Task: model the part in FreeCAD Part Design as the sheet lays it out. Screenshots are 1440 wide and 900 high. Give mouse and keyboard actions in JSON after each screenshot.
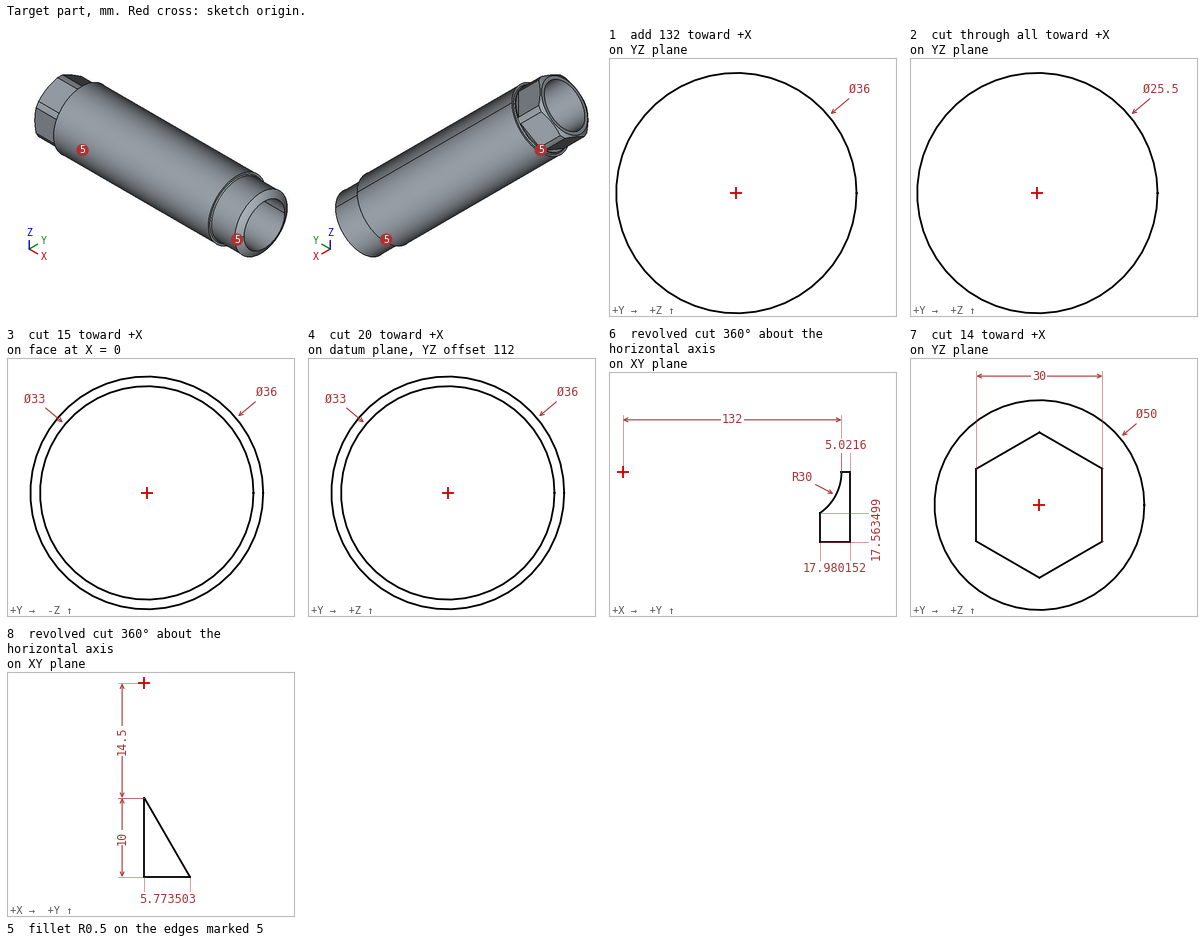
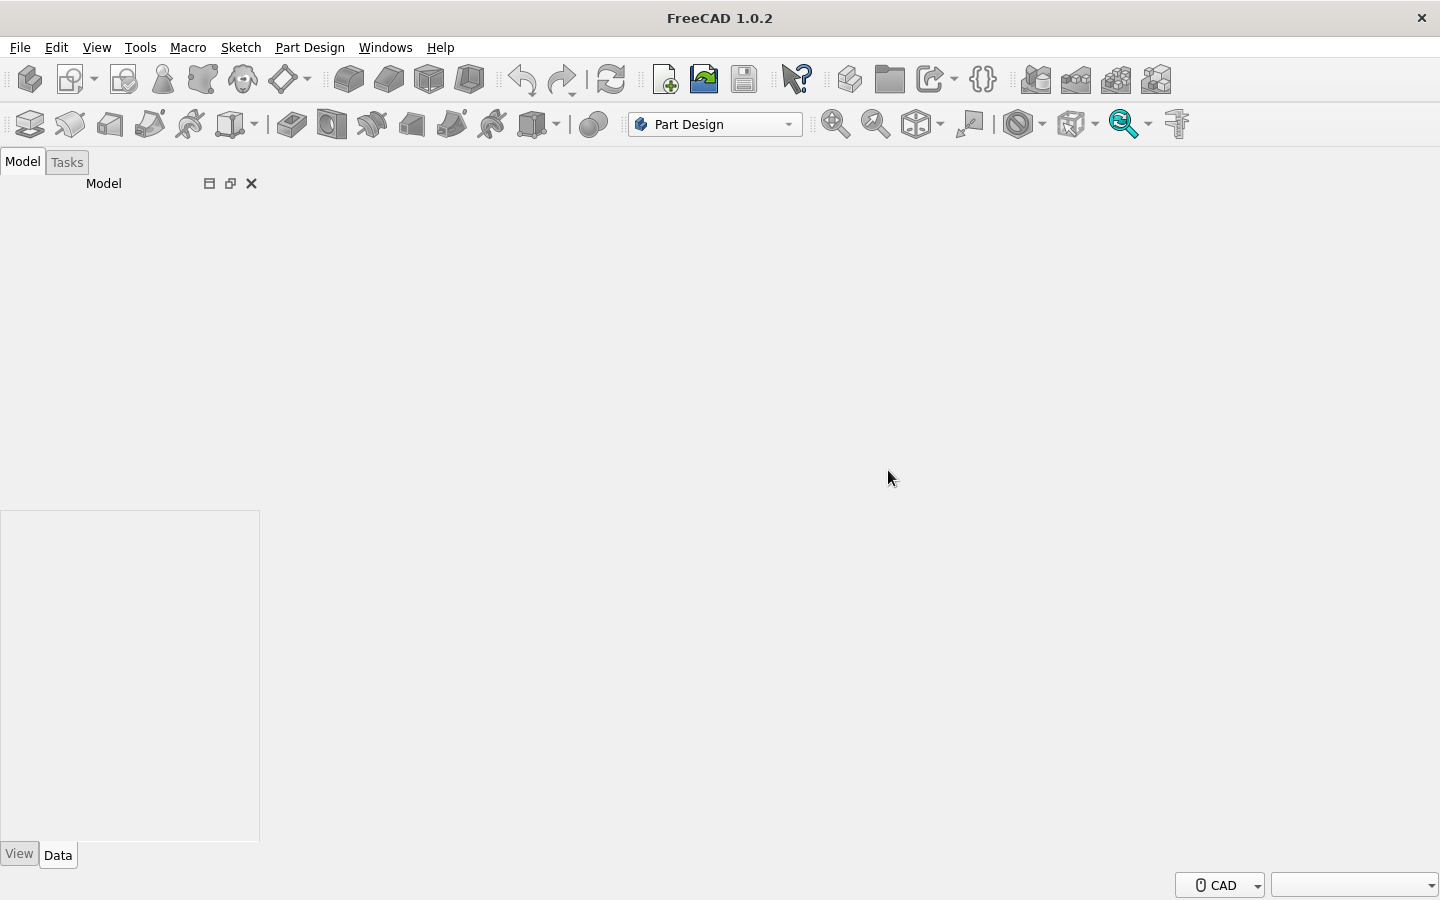
{"action": "left_click", "coordinate": [664, 80]}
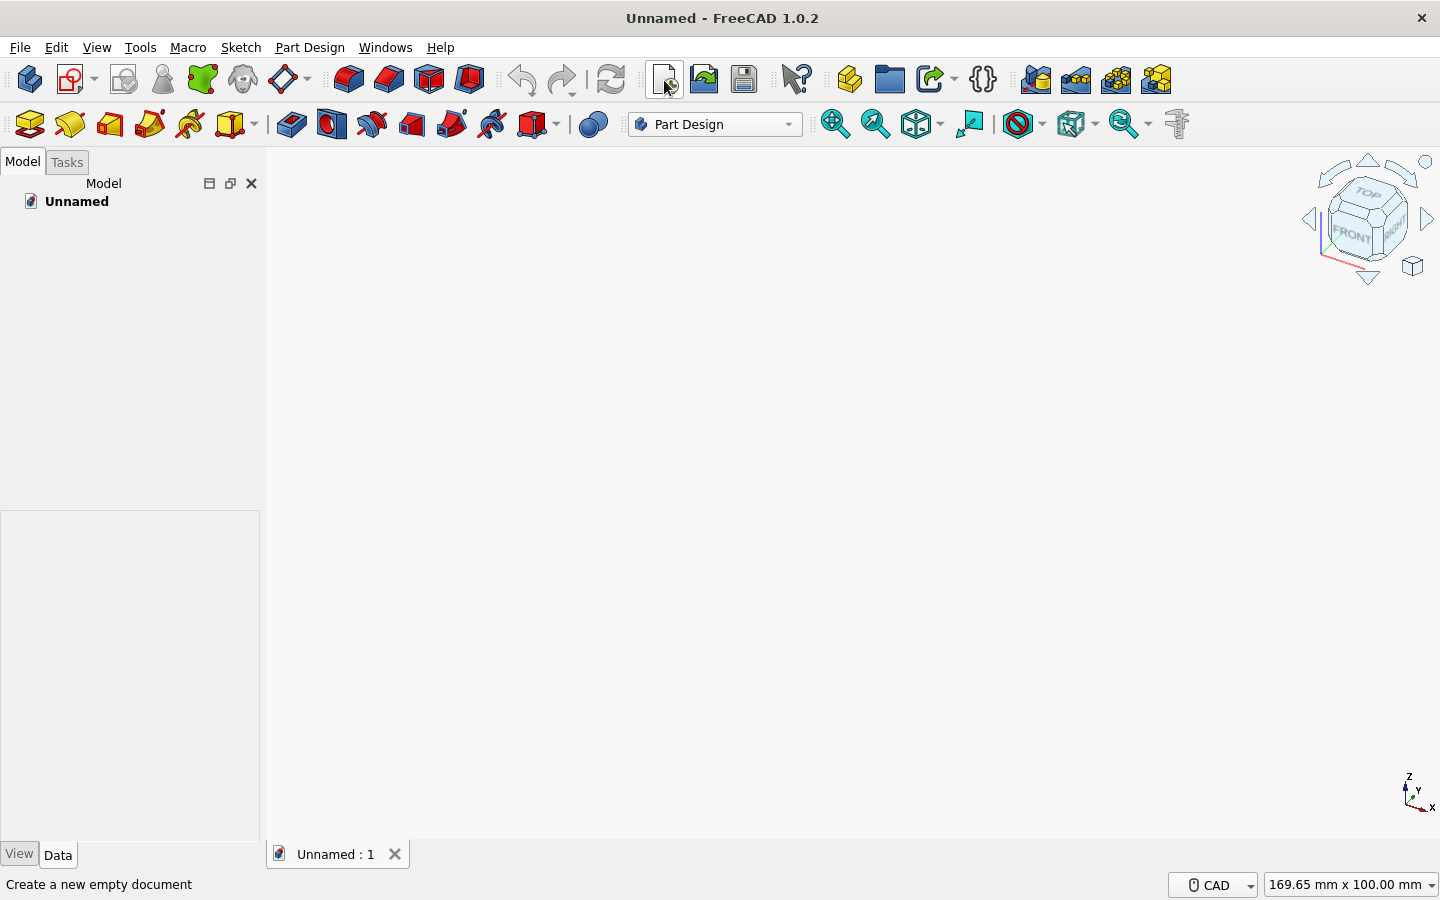
{"action": "left_click", "coordinate": [70, 80]}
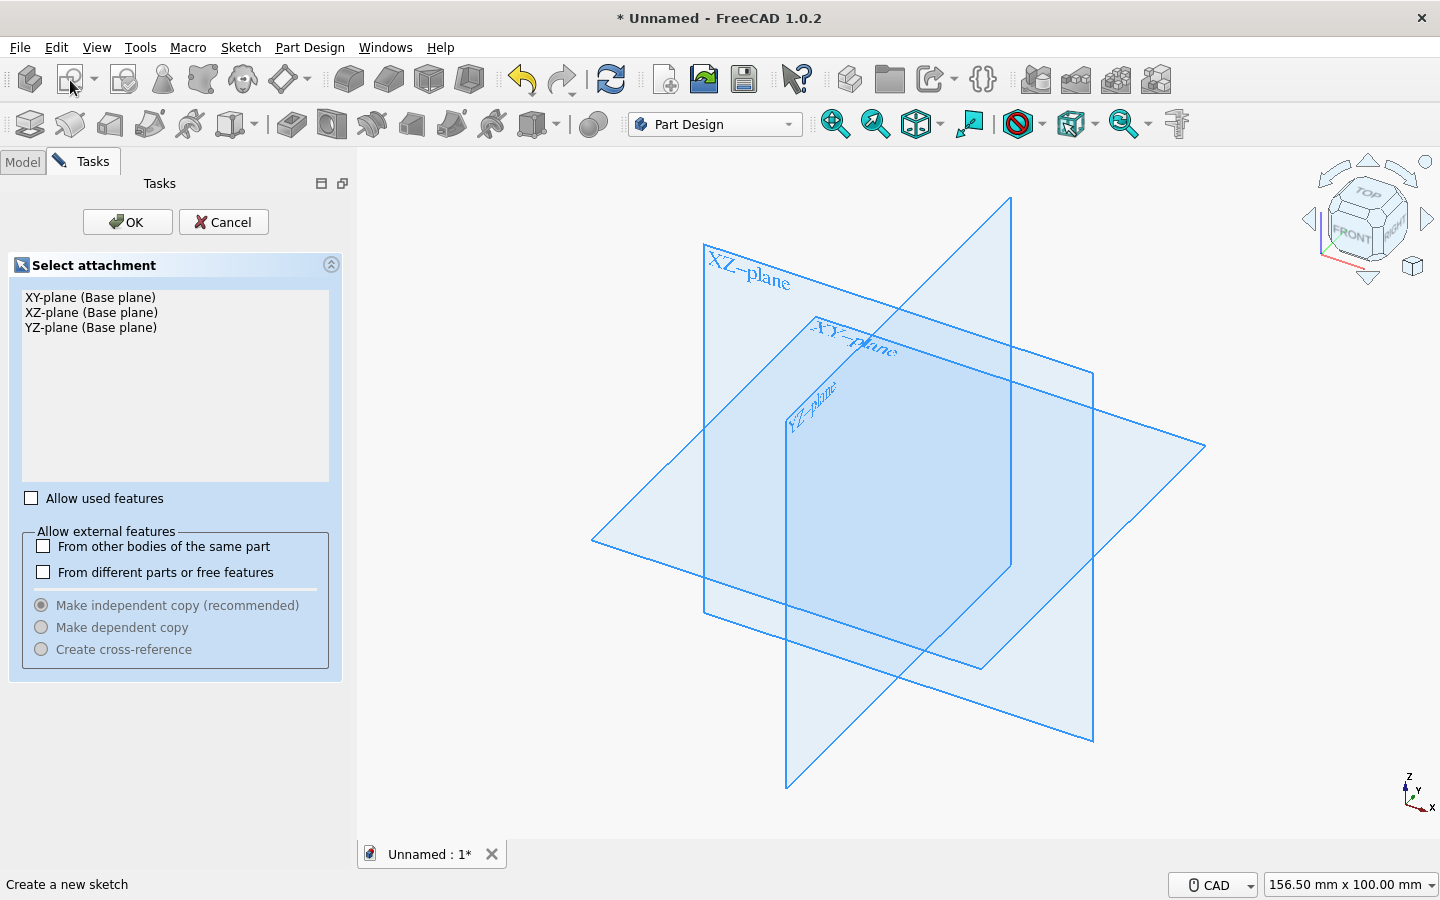
{"action": "left_click", "coordinate": [82, 328]}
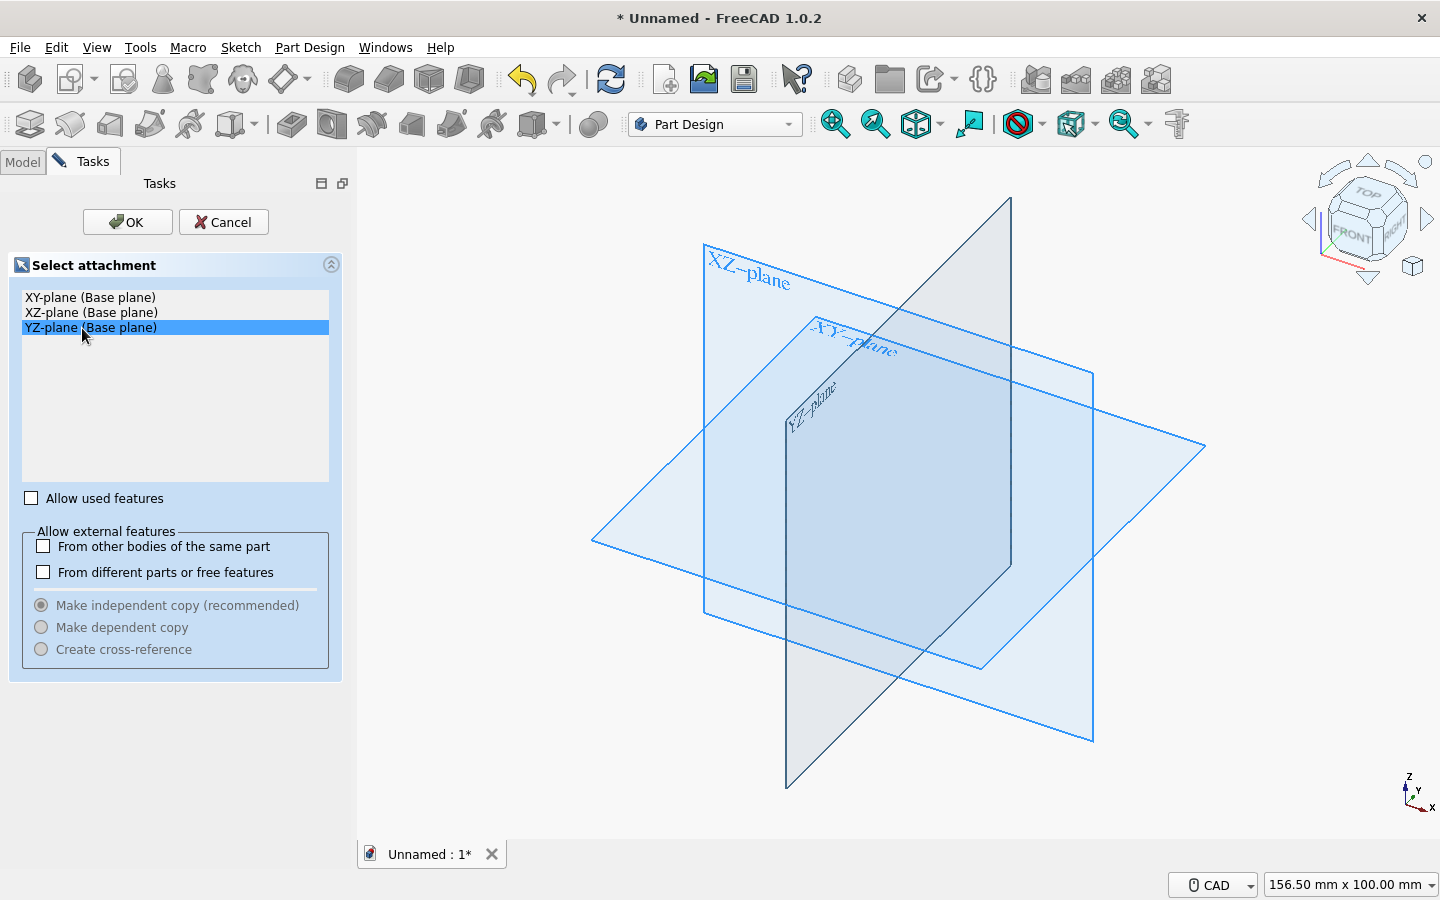
{"action": "left_click", "coordinate": [128, 222]}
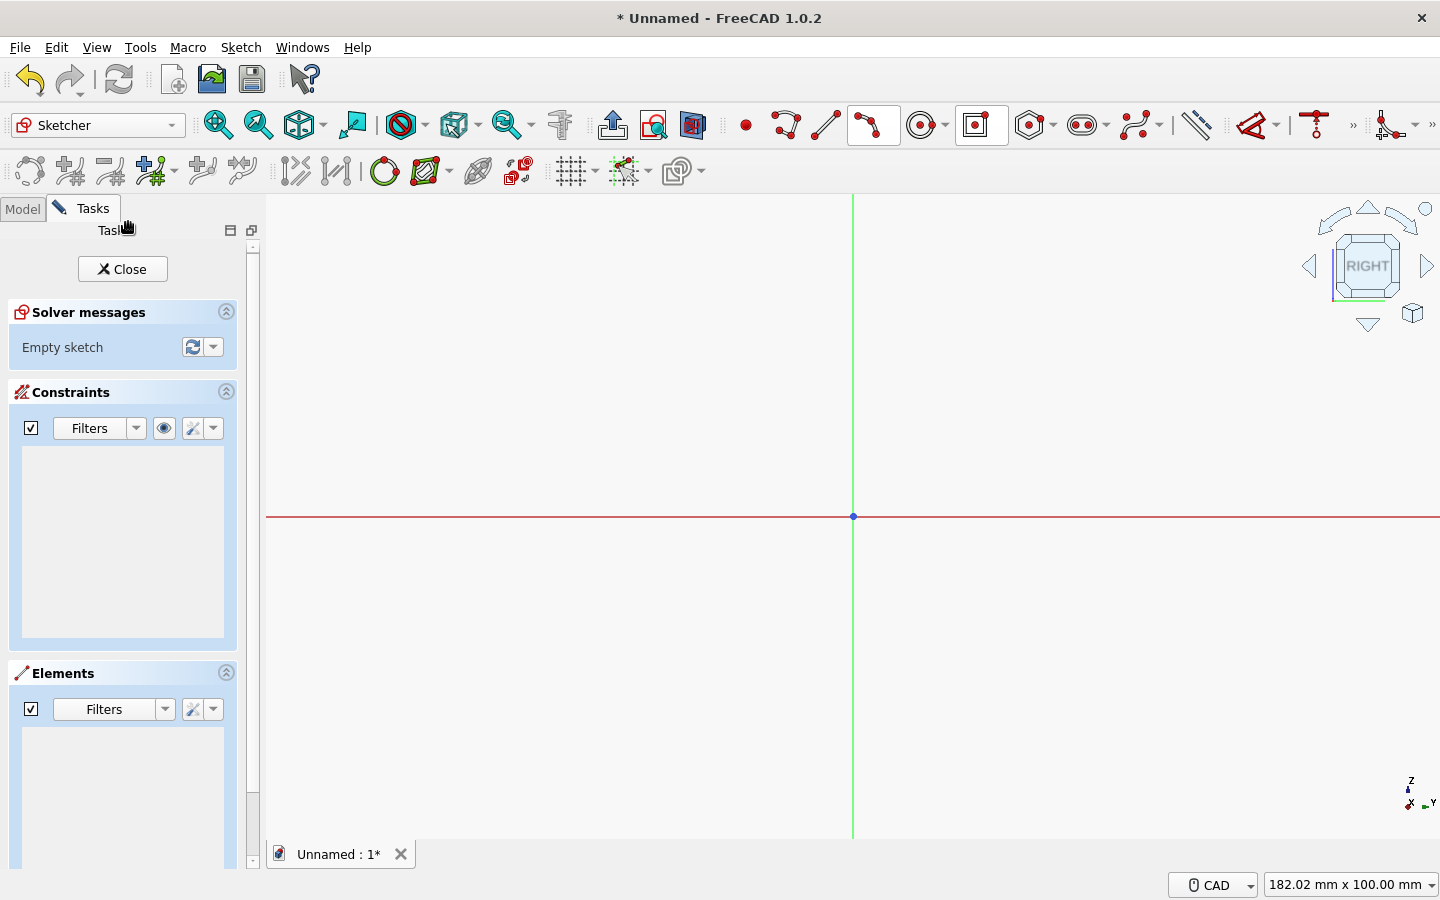
{"action": "scroll", "coordinate": [936, 516], "scroll_direction": "up", "scroll_amount": 3}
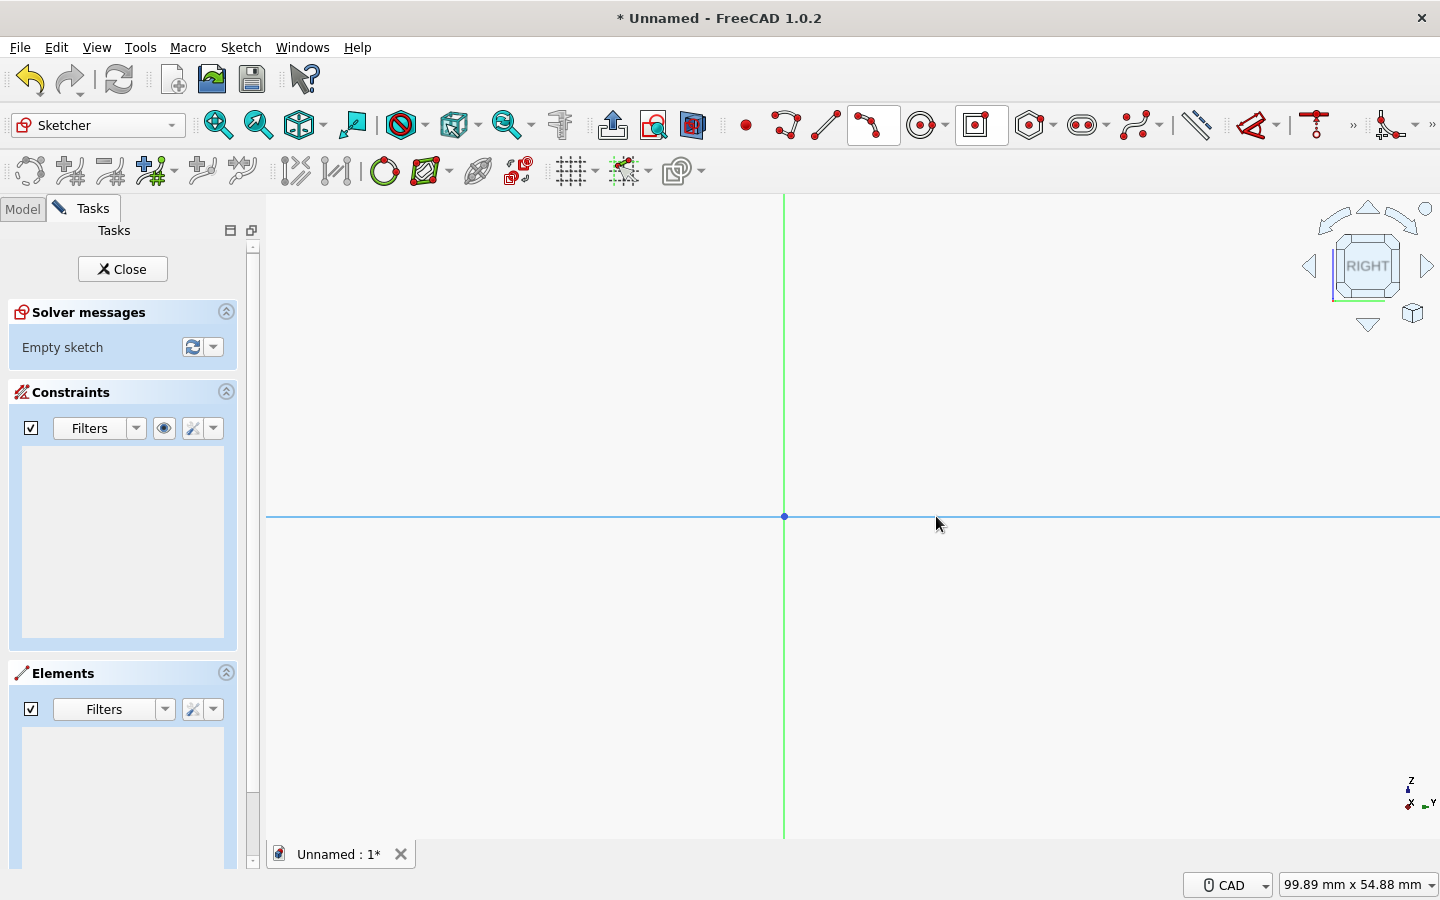
{"action": "left_click", "coordinate": [922, 126]}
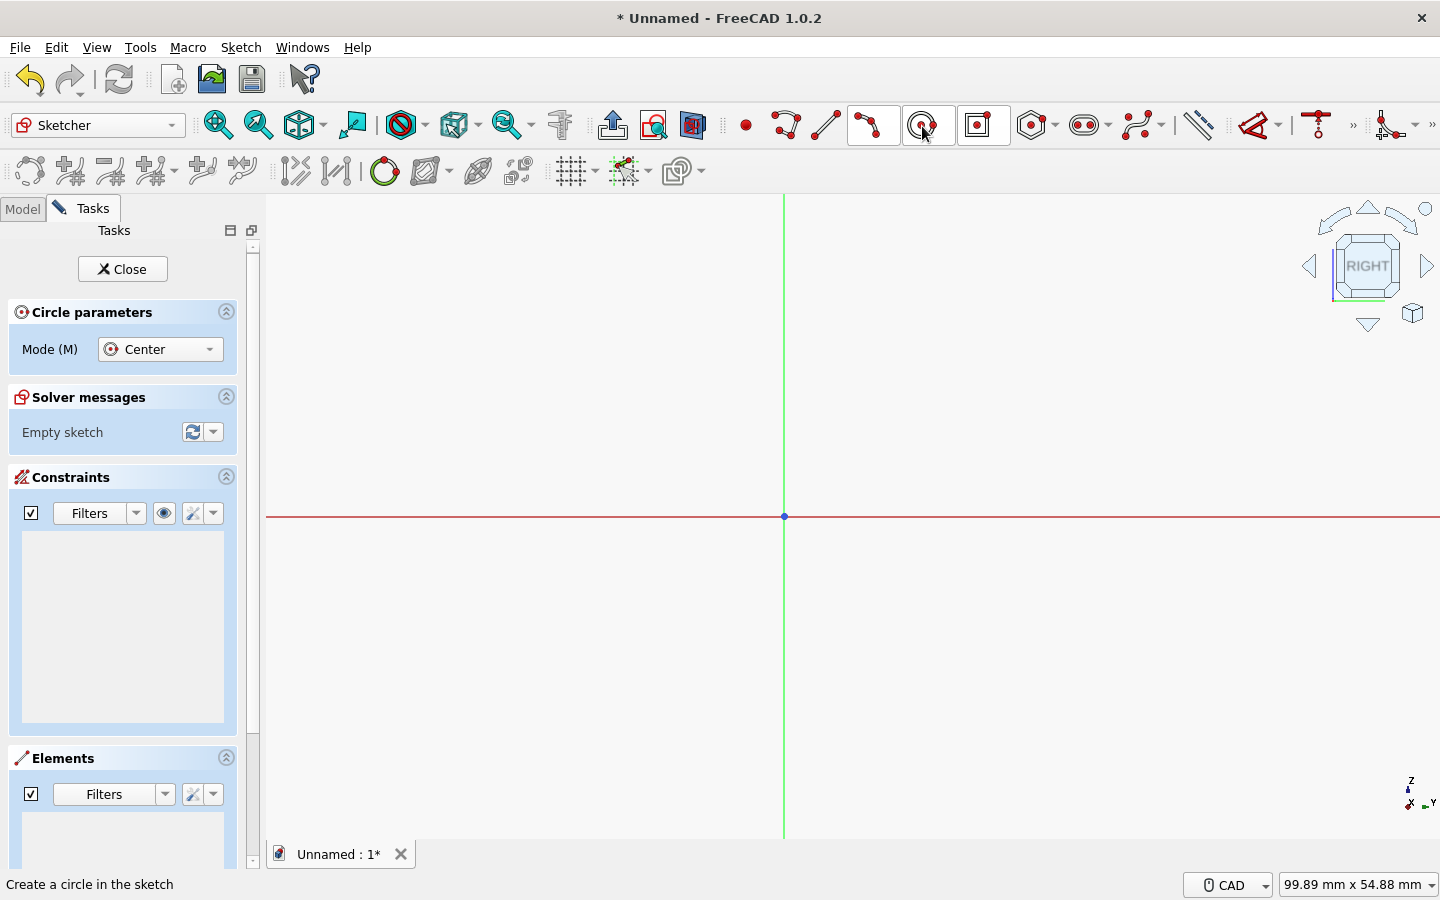
{"action": "left_click", "coordinate": [784, 516]}
{"action": "mouse_move", "coordinate": [934, 367]}